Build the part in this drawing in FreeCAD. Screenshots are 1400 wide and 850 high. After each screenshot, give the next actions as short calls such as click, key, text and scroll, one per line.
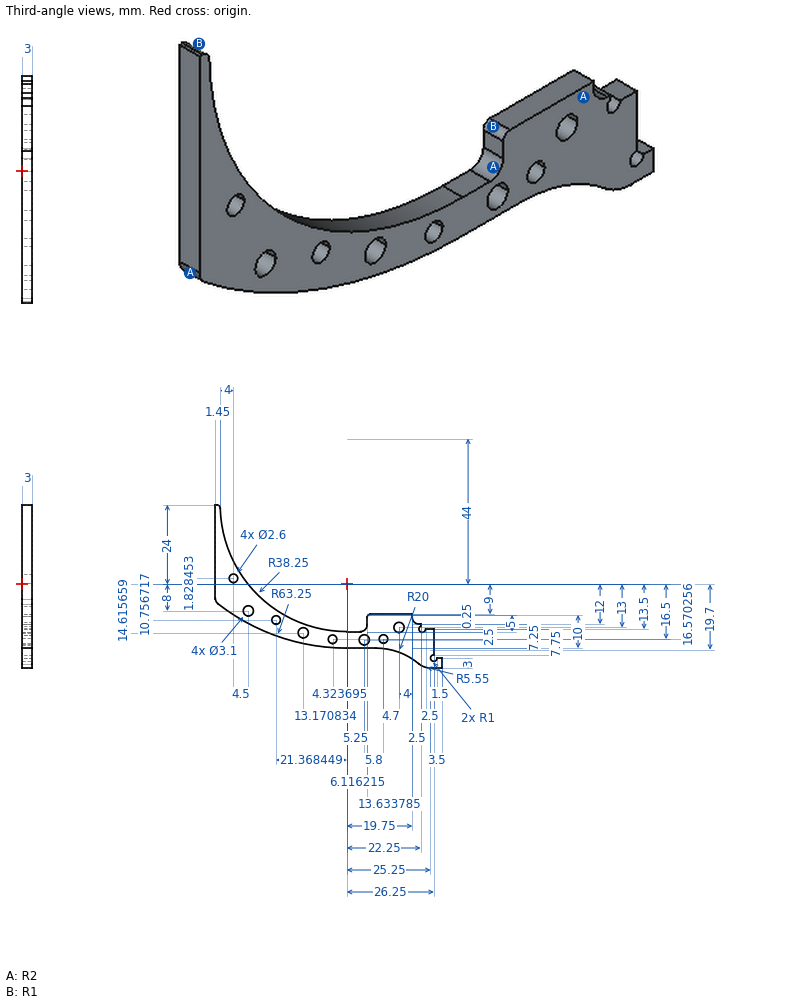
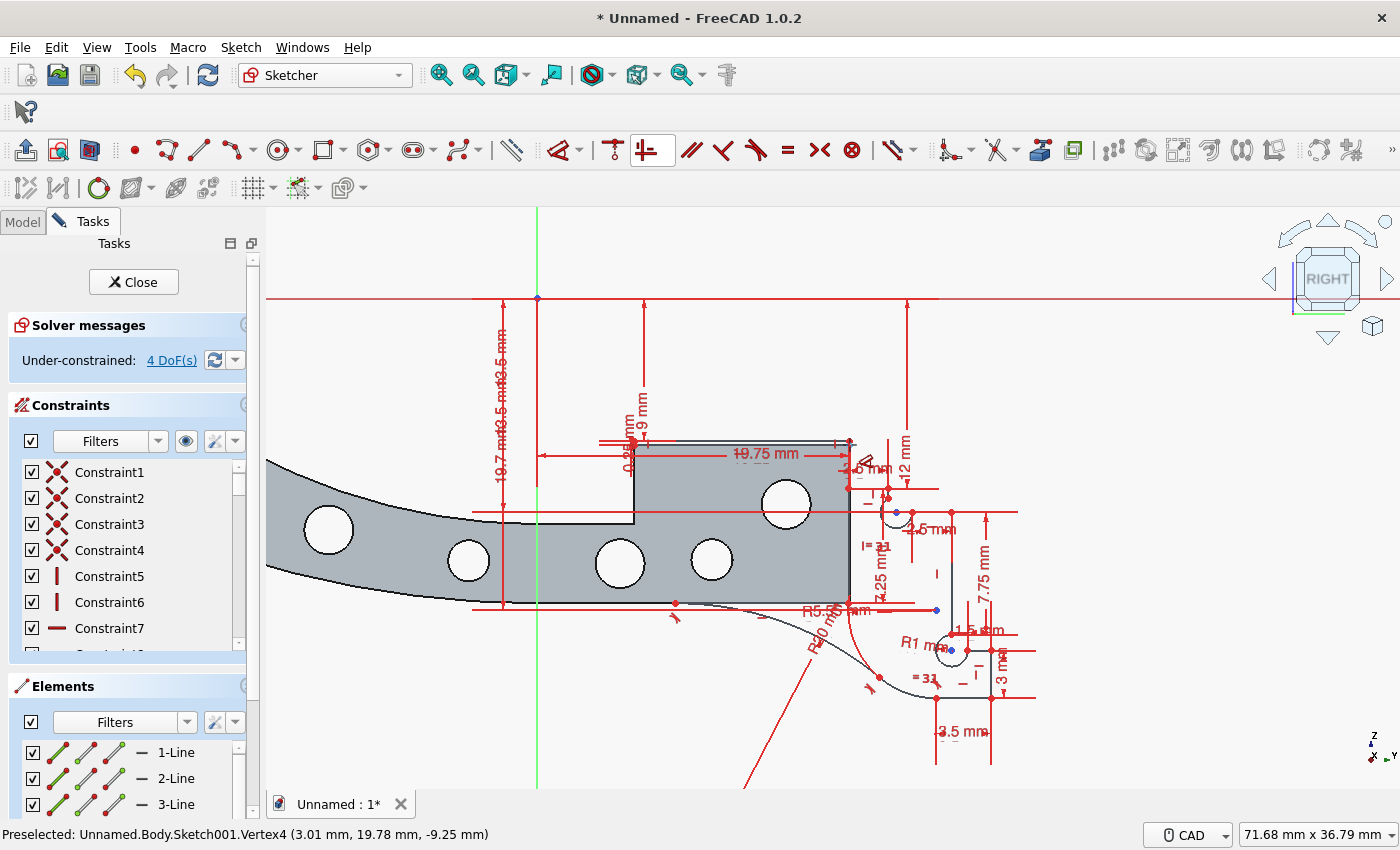
click(936, 698)
click(737, 732)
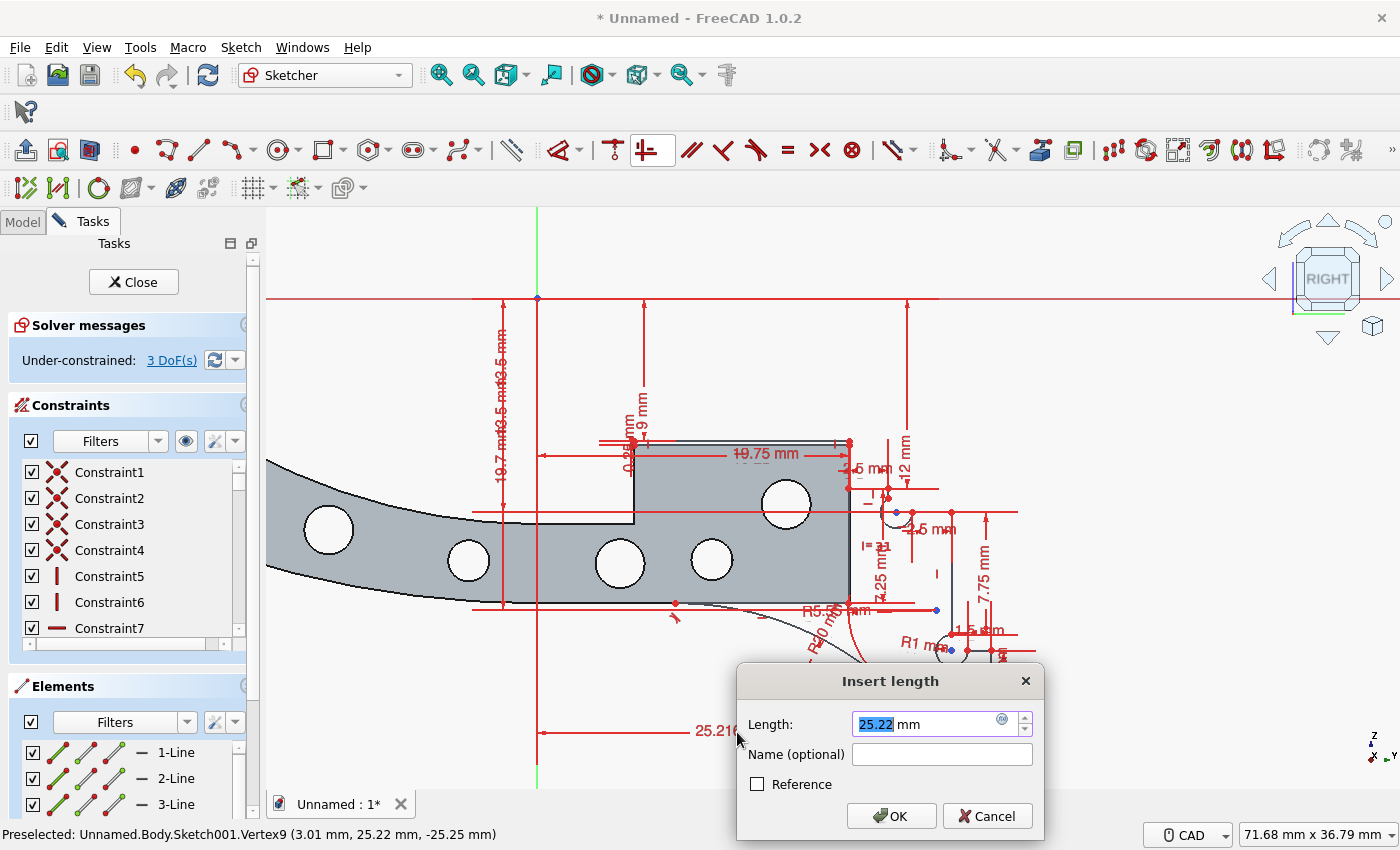
text(25.25)
key(Return)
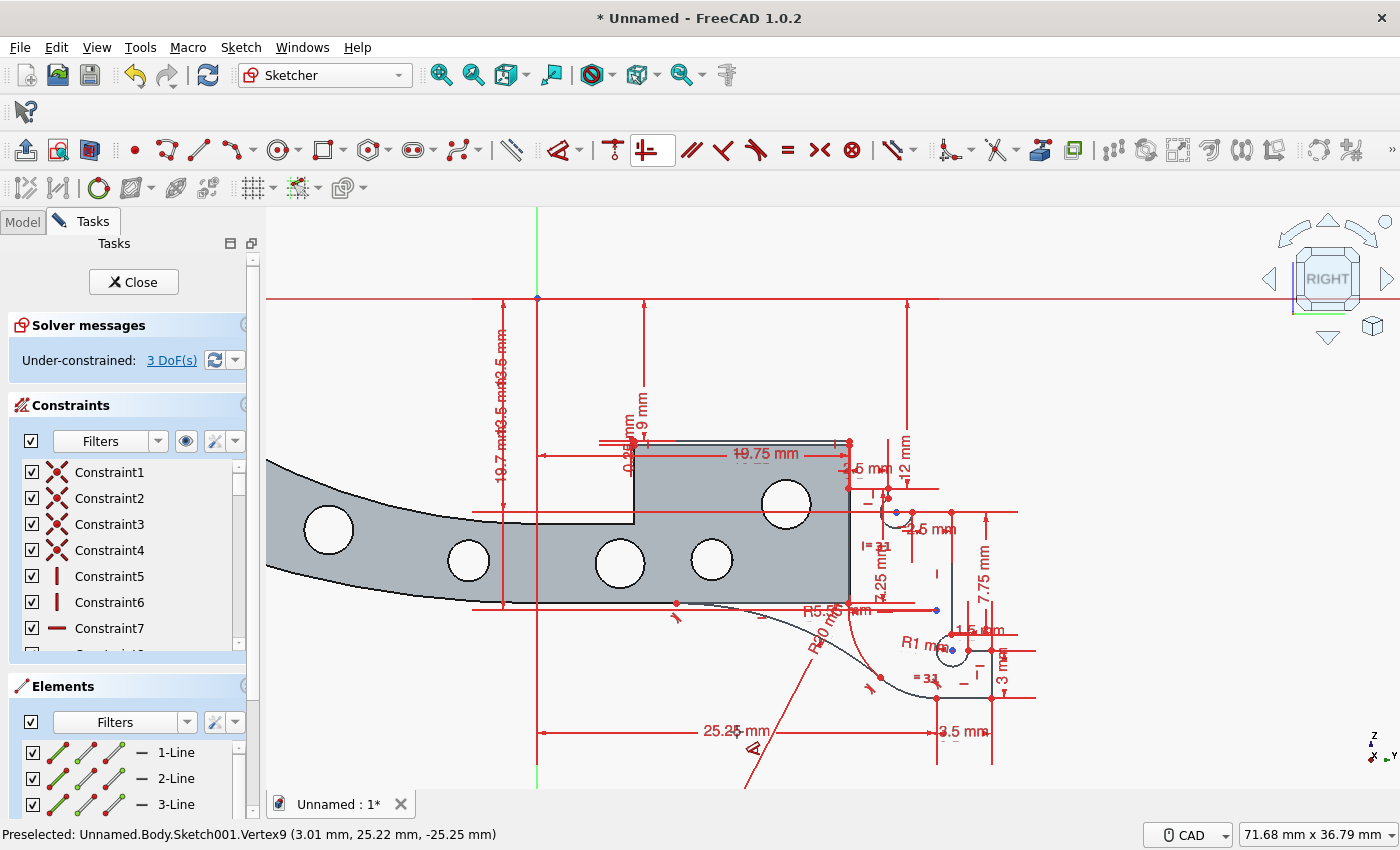
click(952, 635)
click(744, 265)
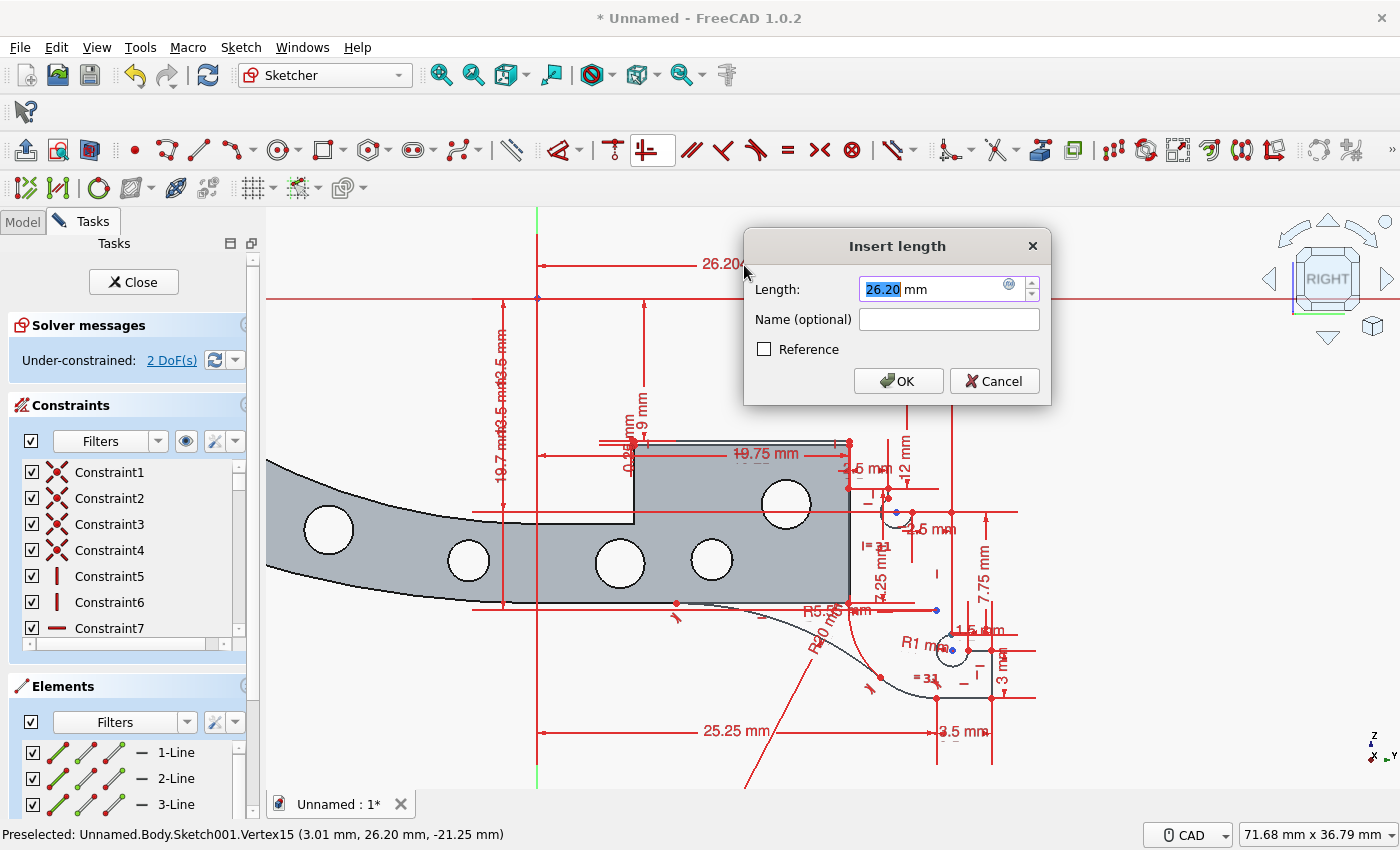
text(26.25)
key(Return)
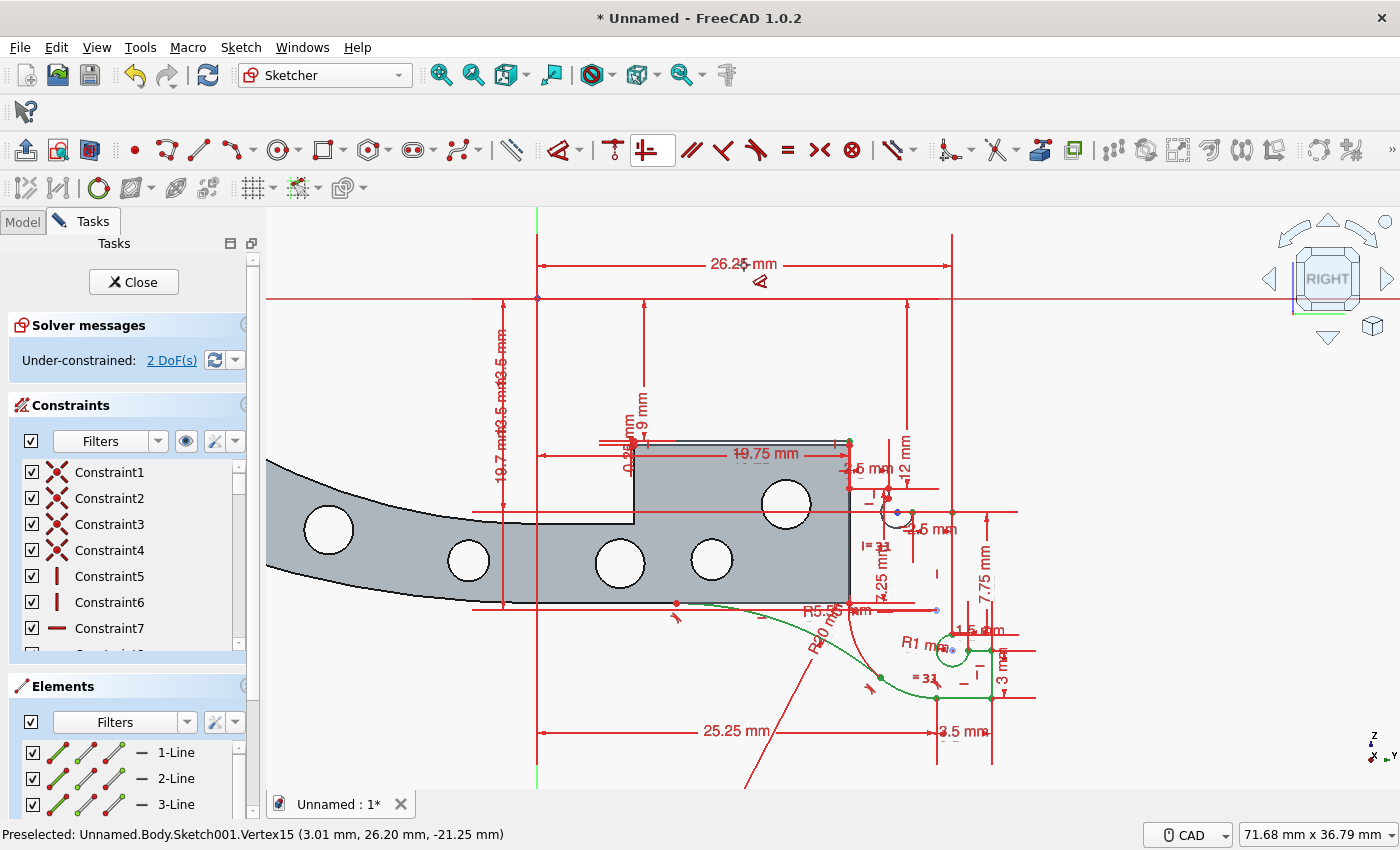
click(889, 499)
click(632, 265)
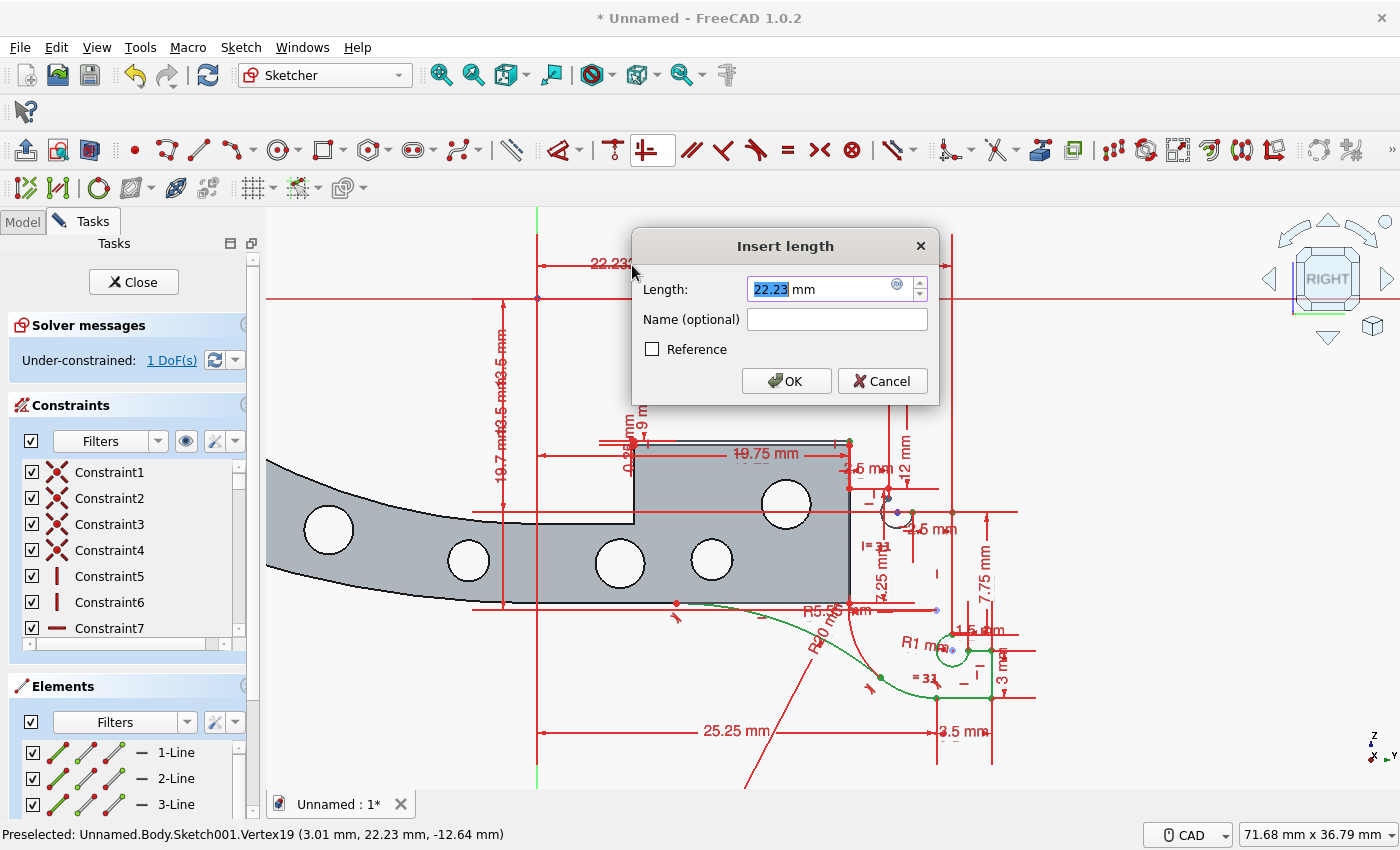
text(22.25)
key(Return)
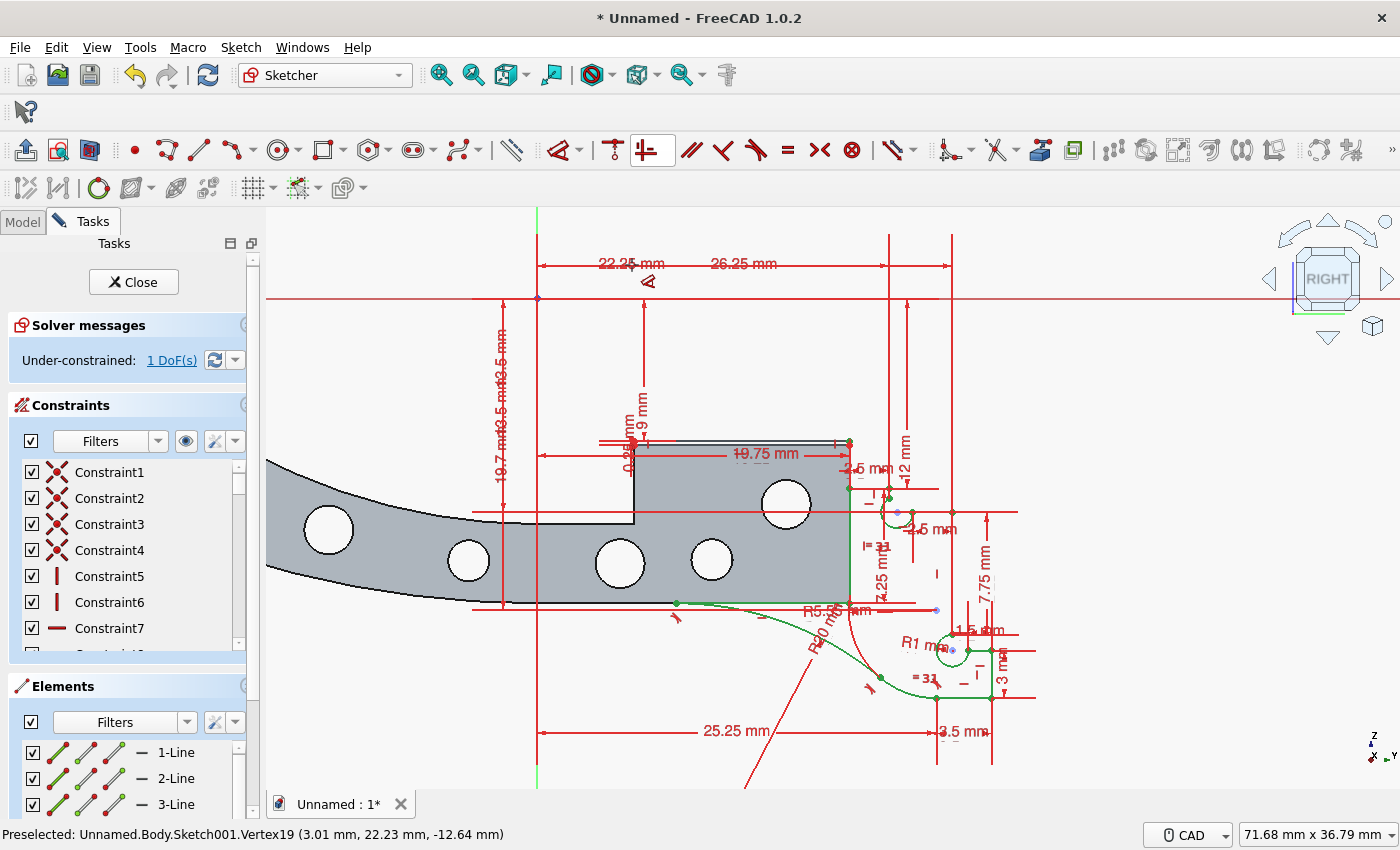
scroll(699, 445, up, 7)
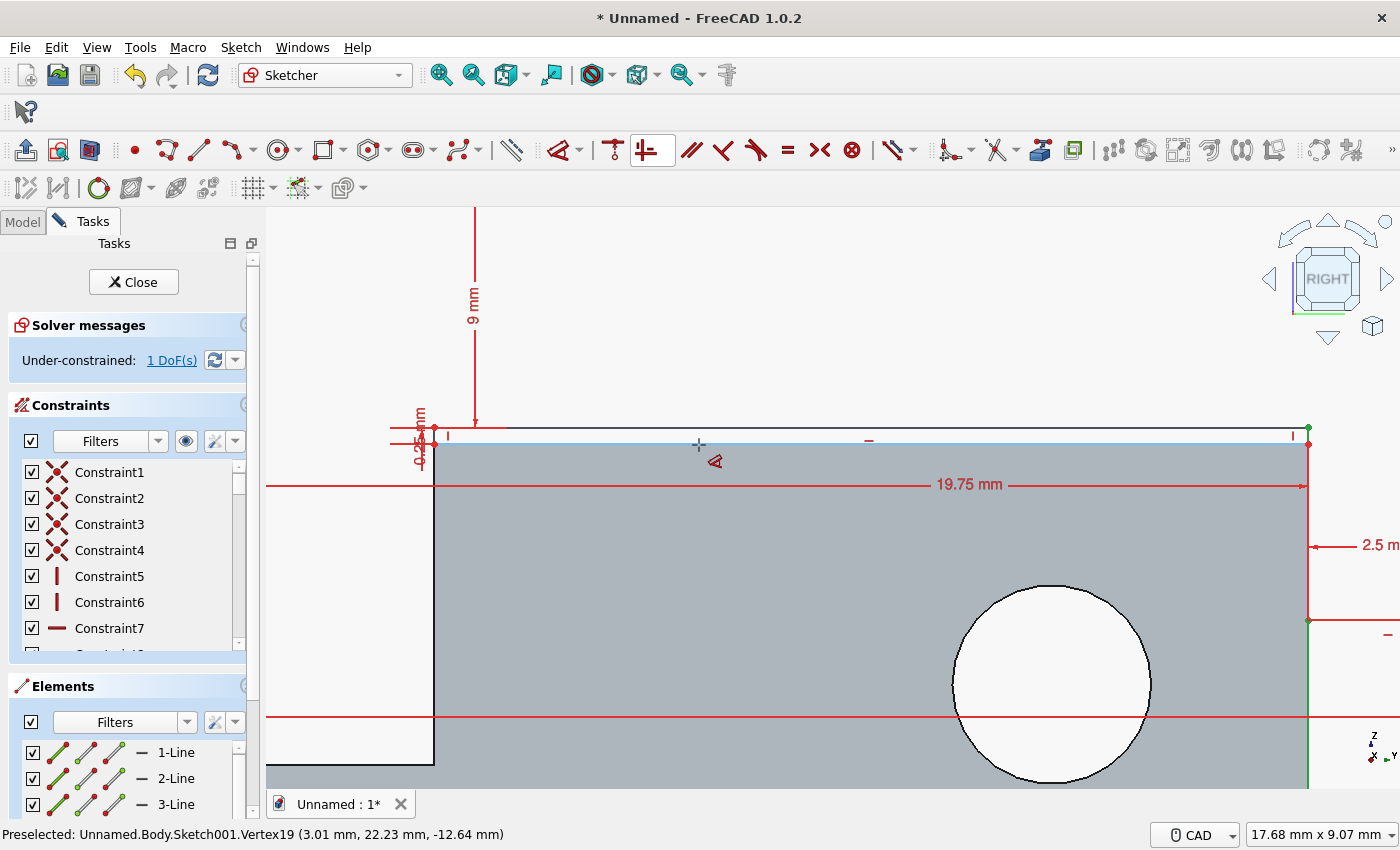
click(697, 444)
click(835, 410)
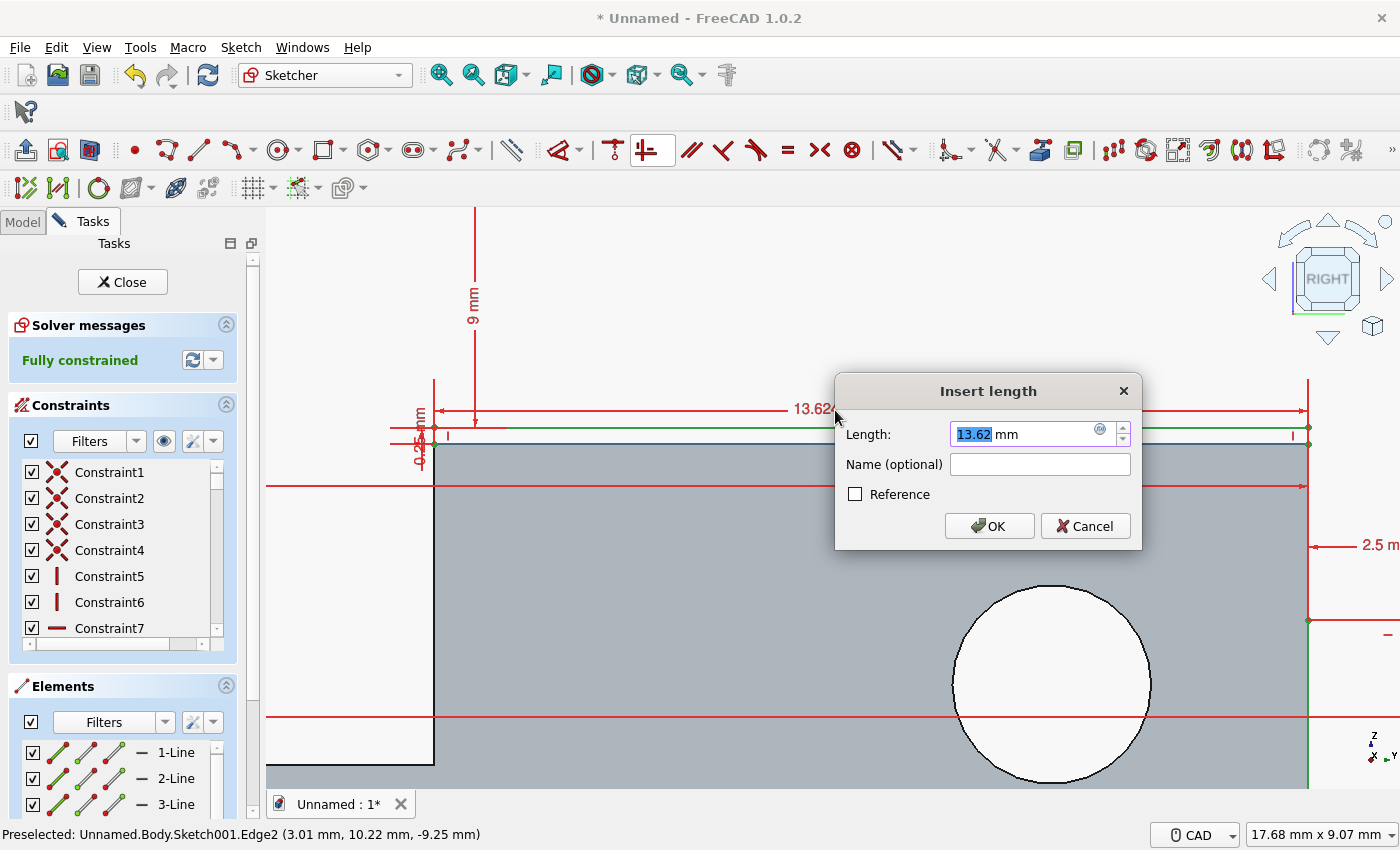
text(13.633785)
key(Return)
key(Escape)